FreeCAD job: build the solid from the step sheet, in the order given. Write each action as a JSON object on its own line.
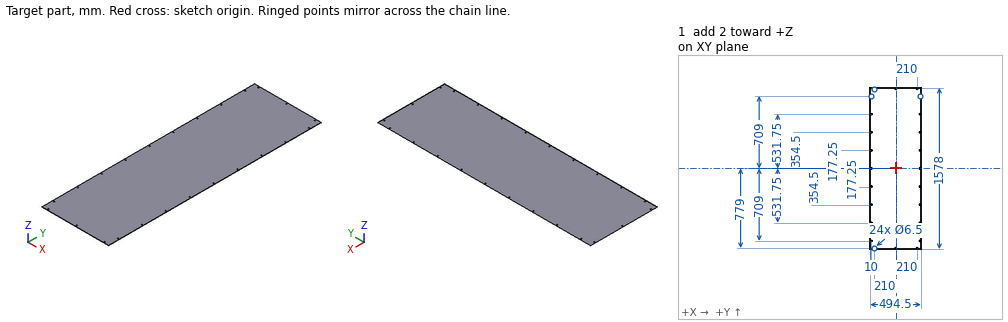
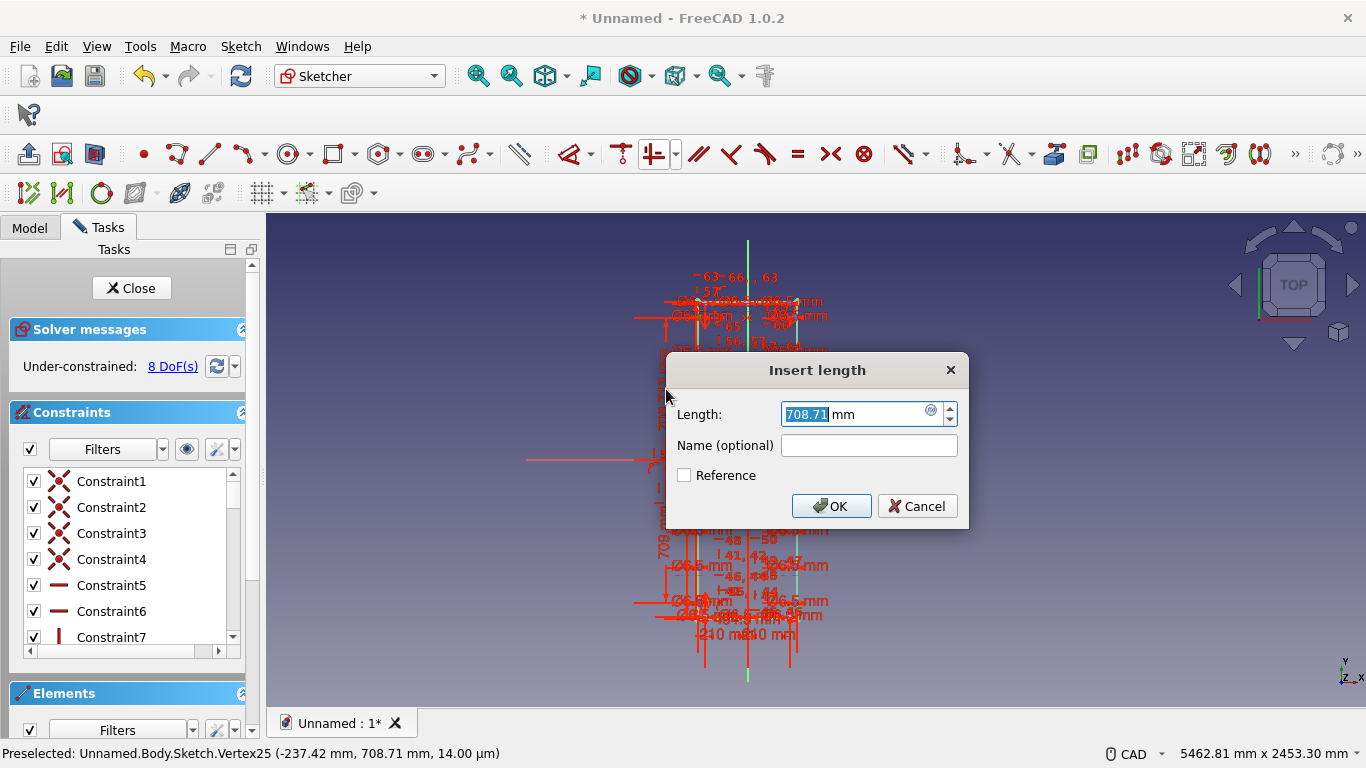
{"action": "type", "text": "709"}
{"action": "key", "text": "Return"}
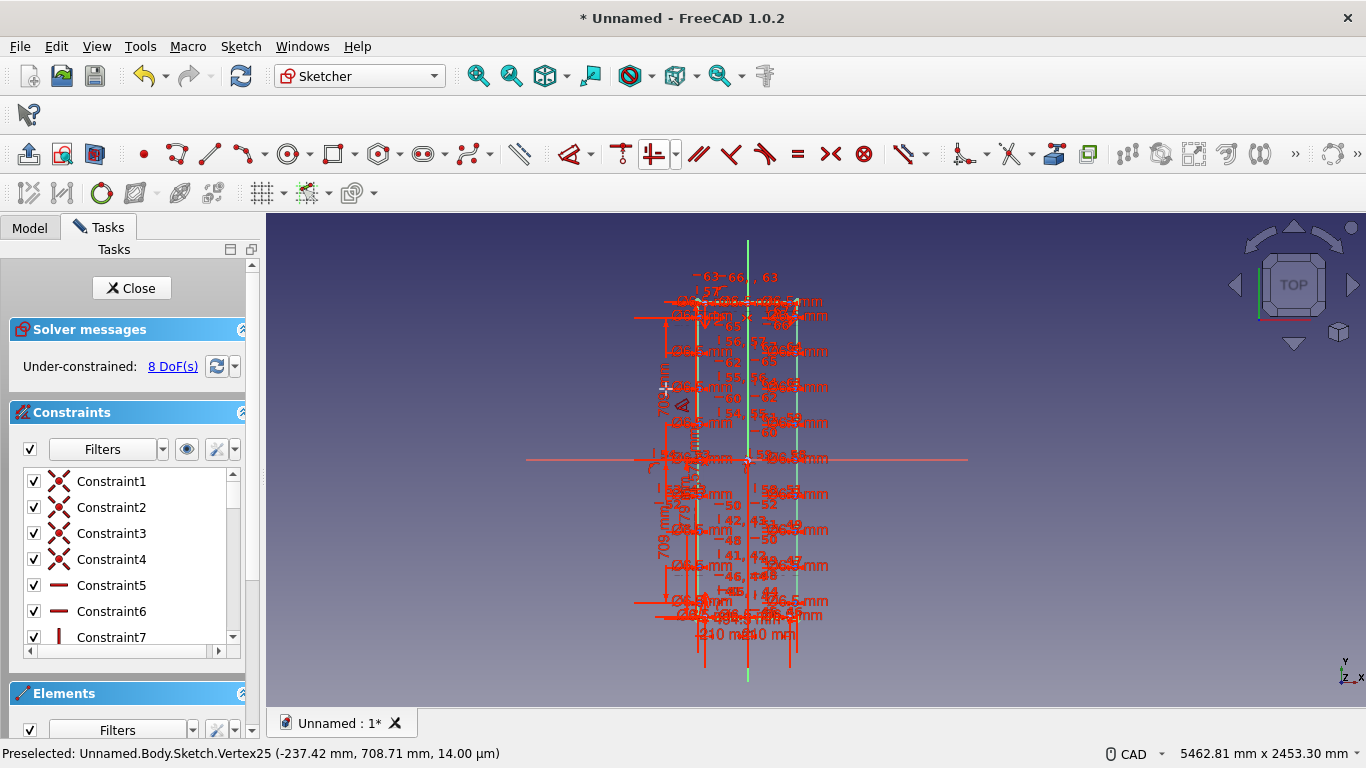
{"action": "scroll", "coordinate": [790, 304], "scroll_direction": "up", "scroll_amount": 3}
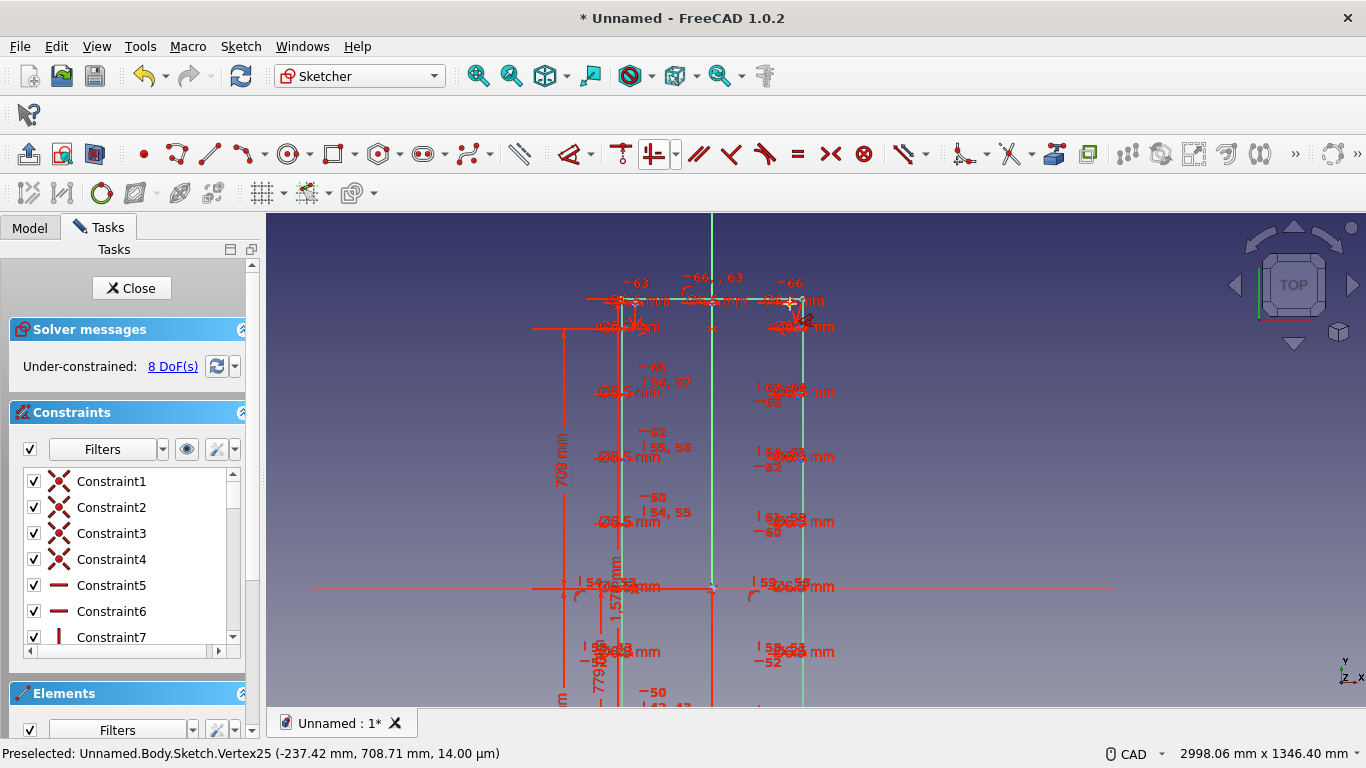
{"action": "left_click", "coordinate": [789, 303]}
{"action": "left_click", "coordinate": [751, 269]}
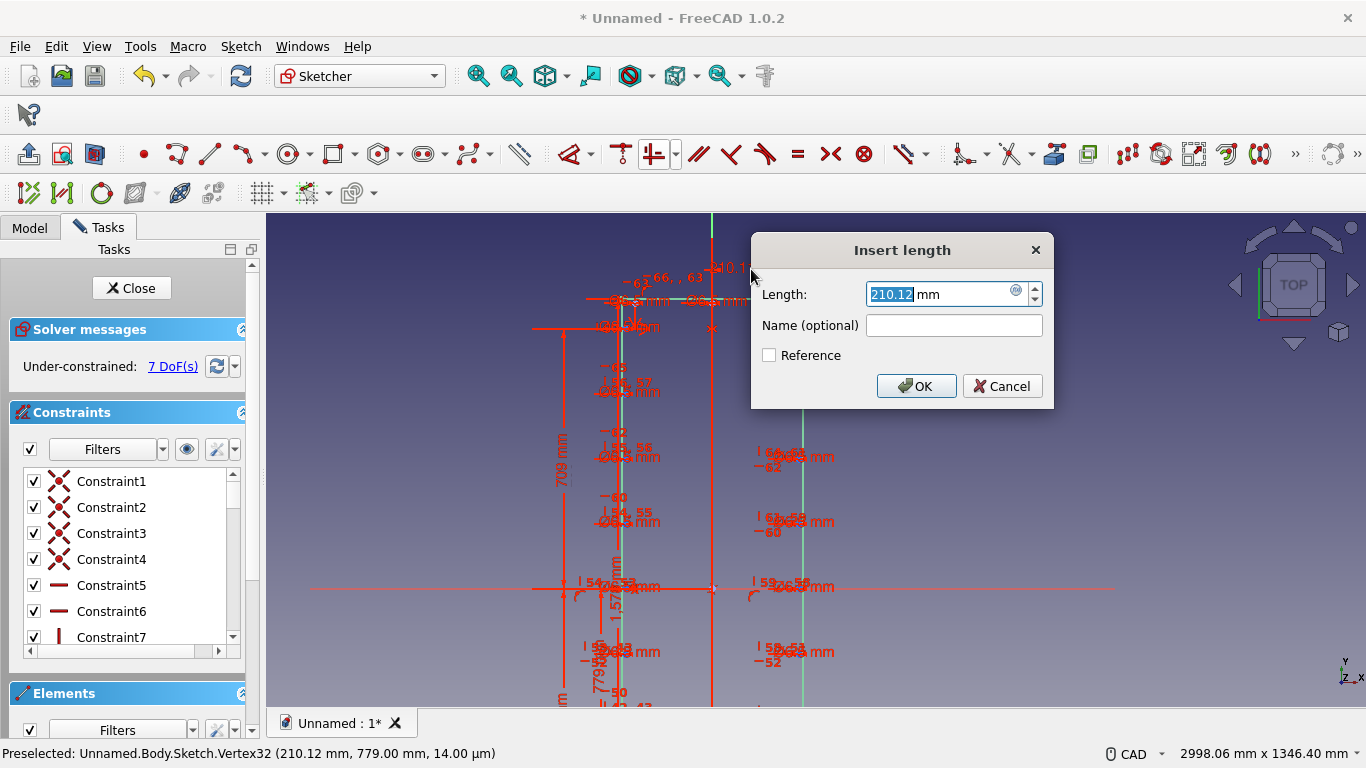
{"action": "type", "text": "210"}
{"action": "key", "text": "Return"}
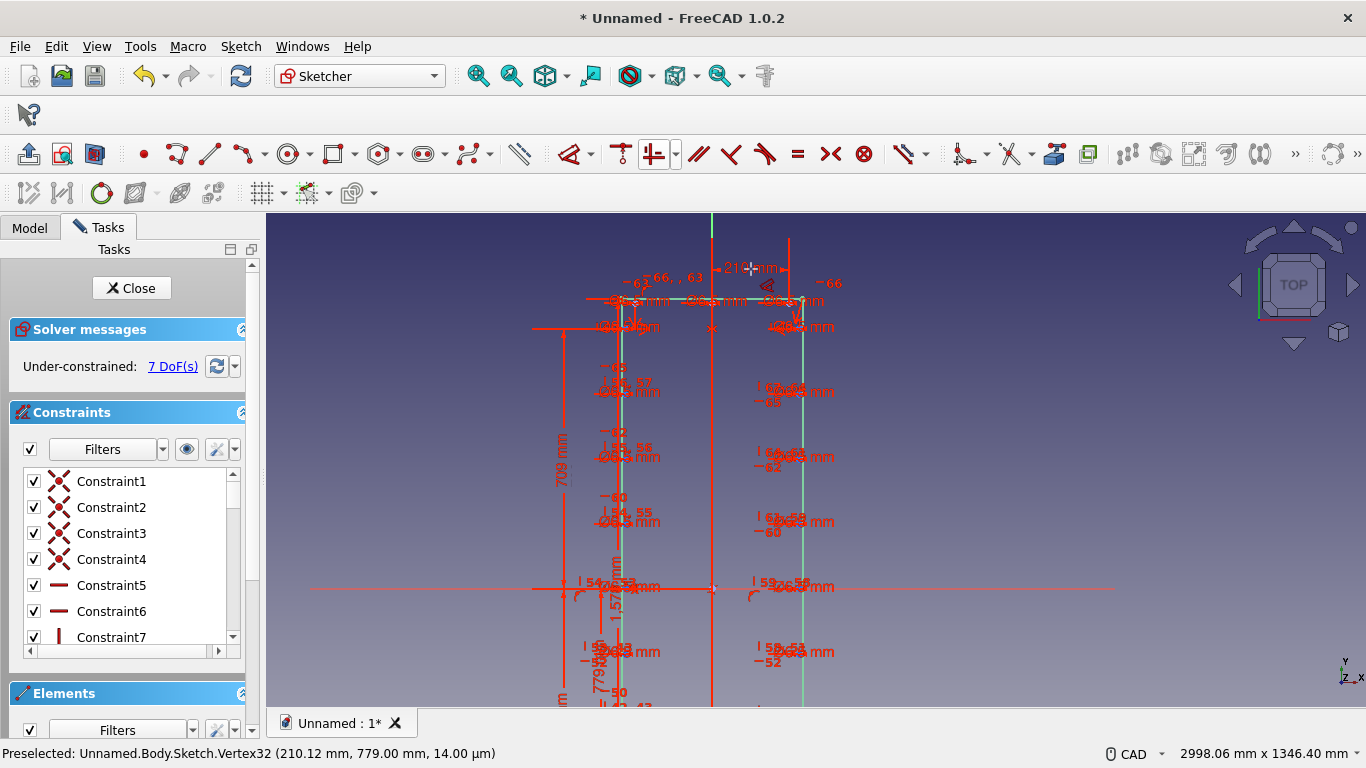
{"action": "scroll", "coordinate": [790, 303], "scroll_direction": "down", "scroll_amount": 3}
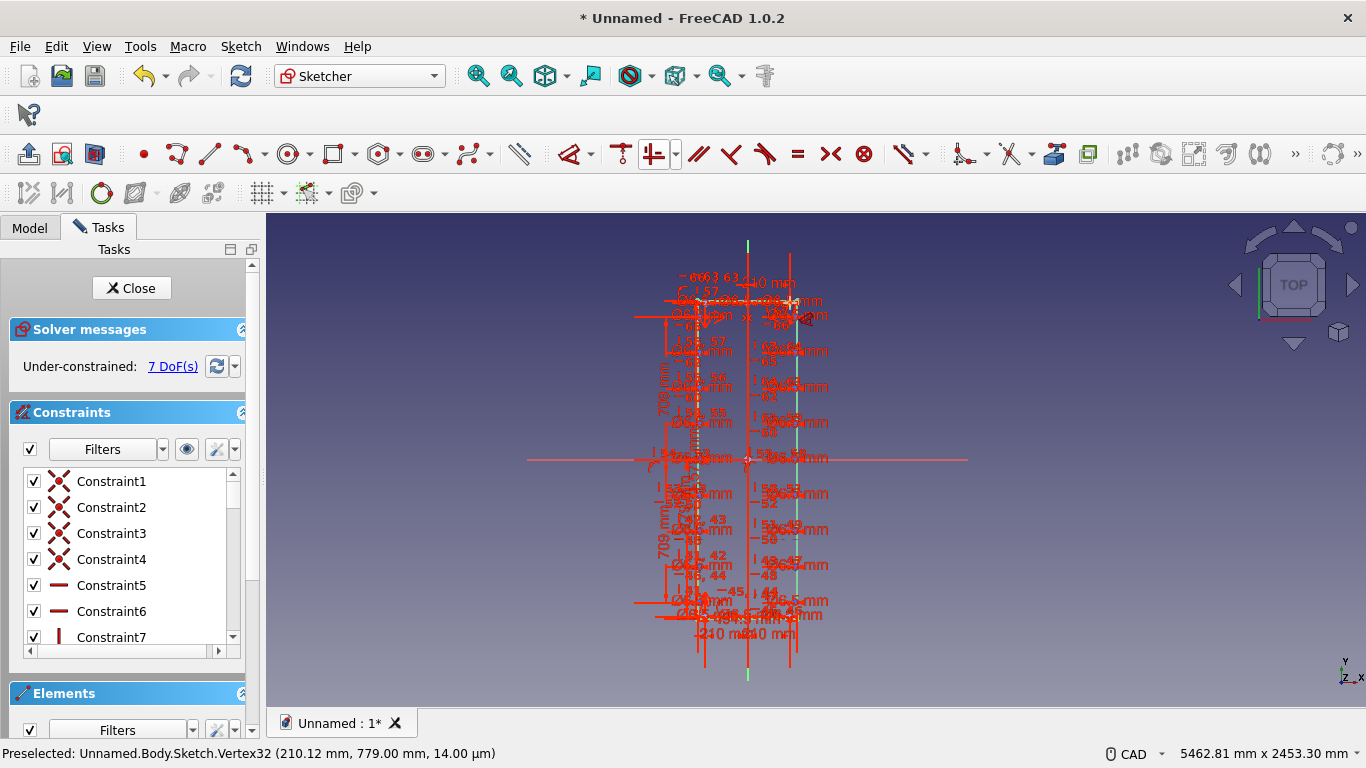
{"action": "scroll", "coordinate": [698, 619], "scroll_direction": "up", "scroll_amount": 15}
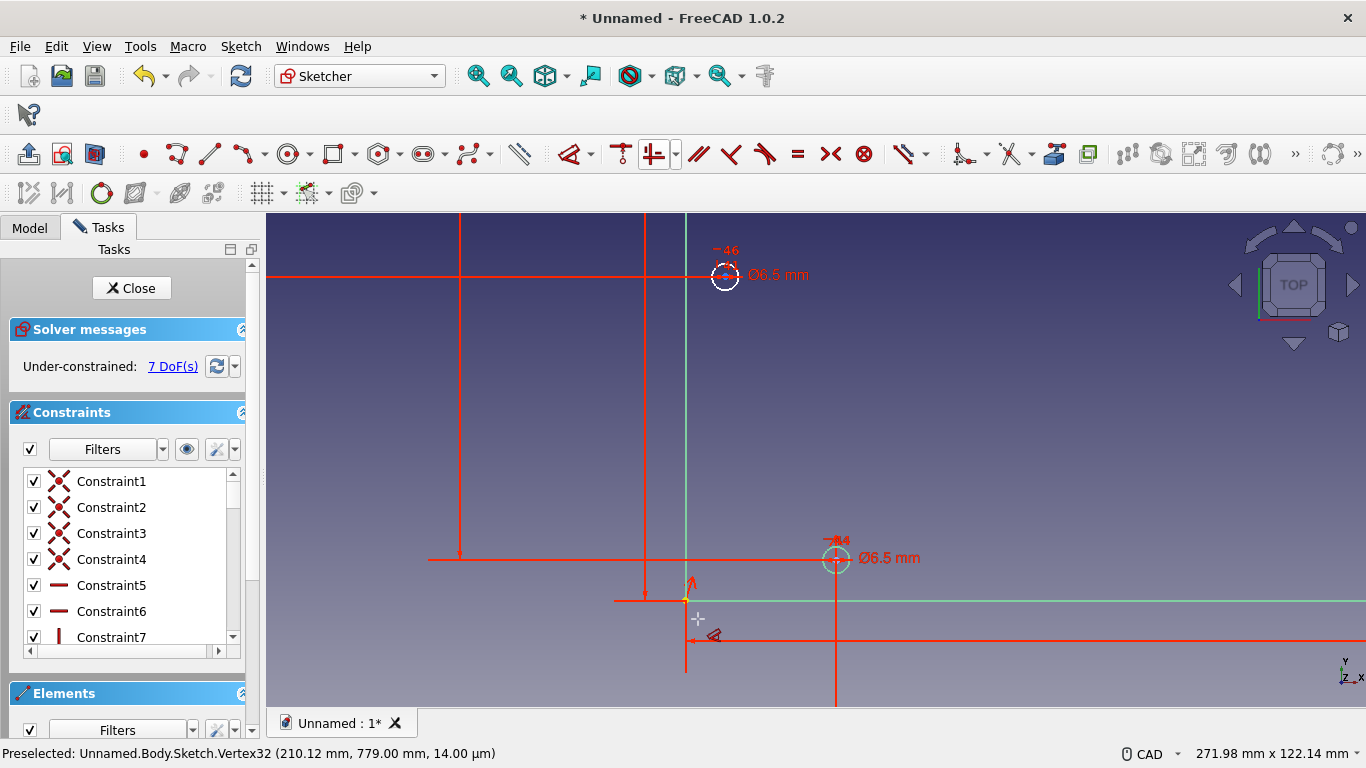
{"action": "left_click", "coordinate": [686, 601]}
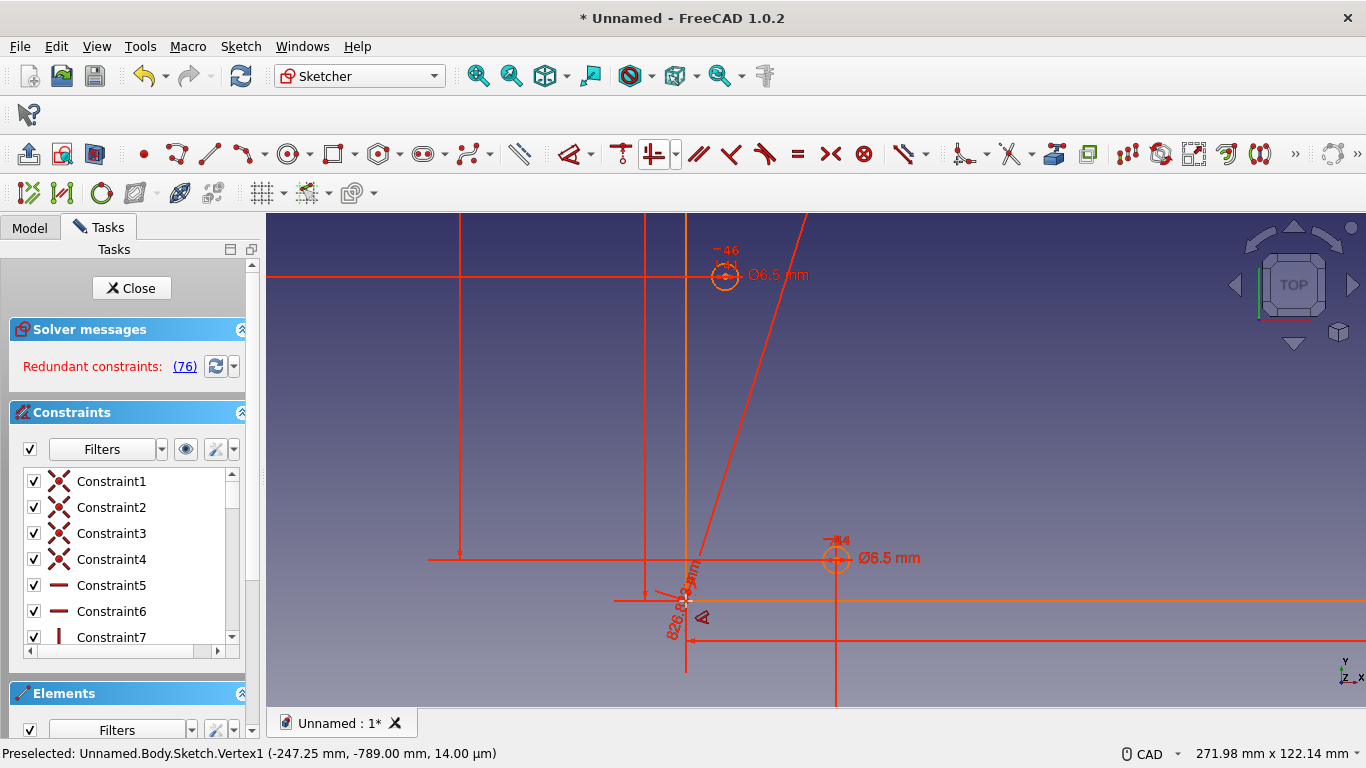
{"action": "left_click", "coordinate": [725, 277]}
{"action": "left_click", "coordinate": [705, 635]}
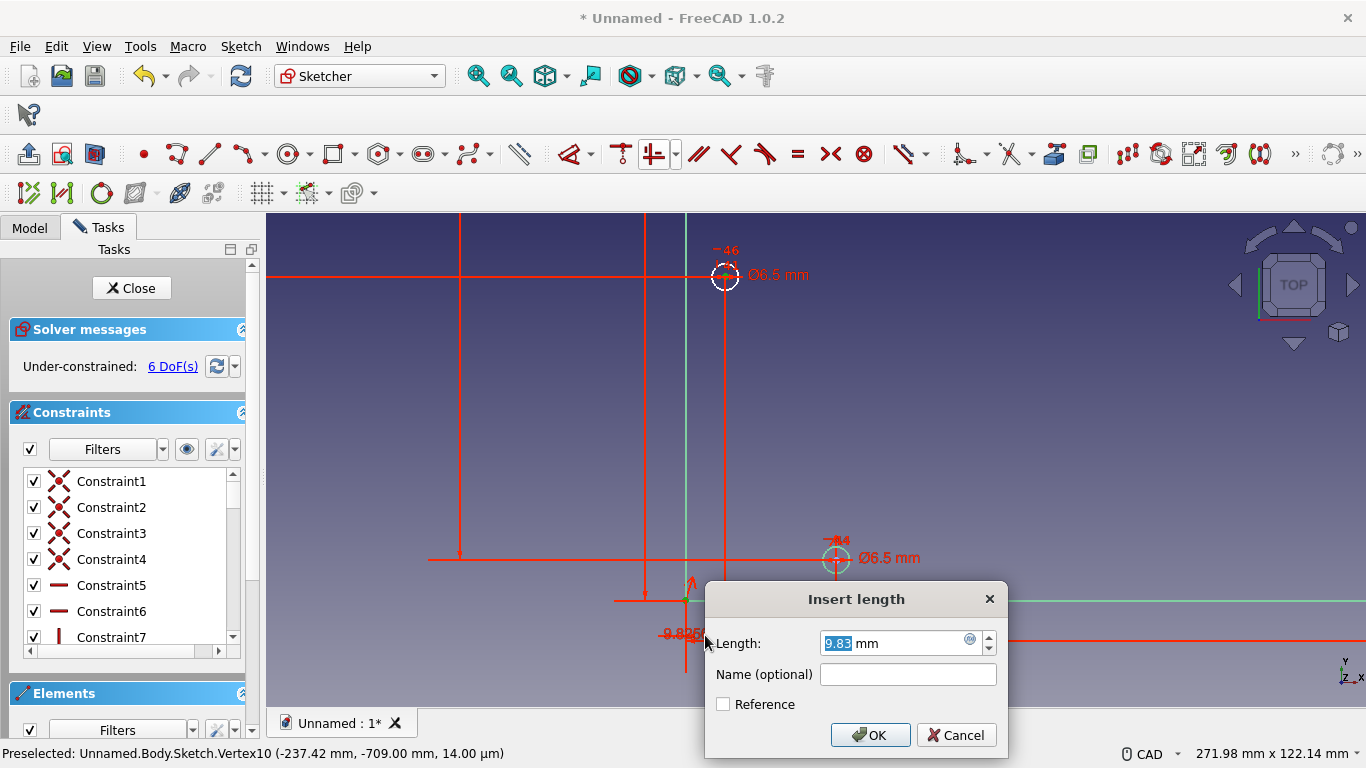
{"action": "type", "text": "10"}
{"action": "key", "text": "Return"}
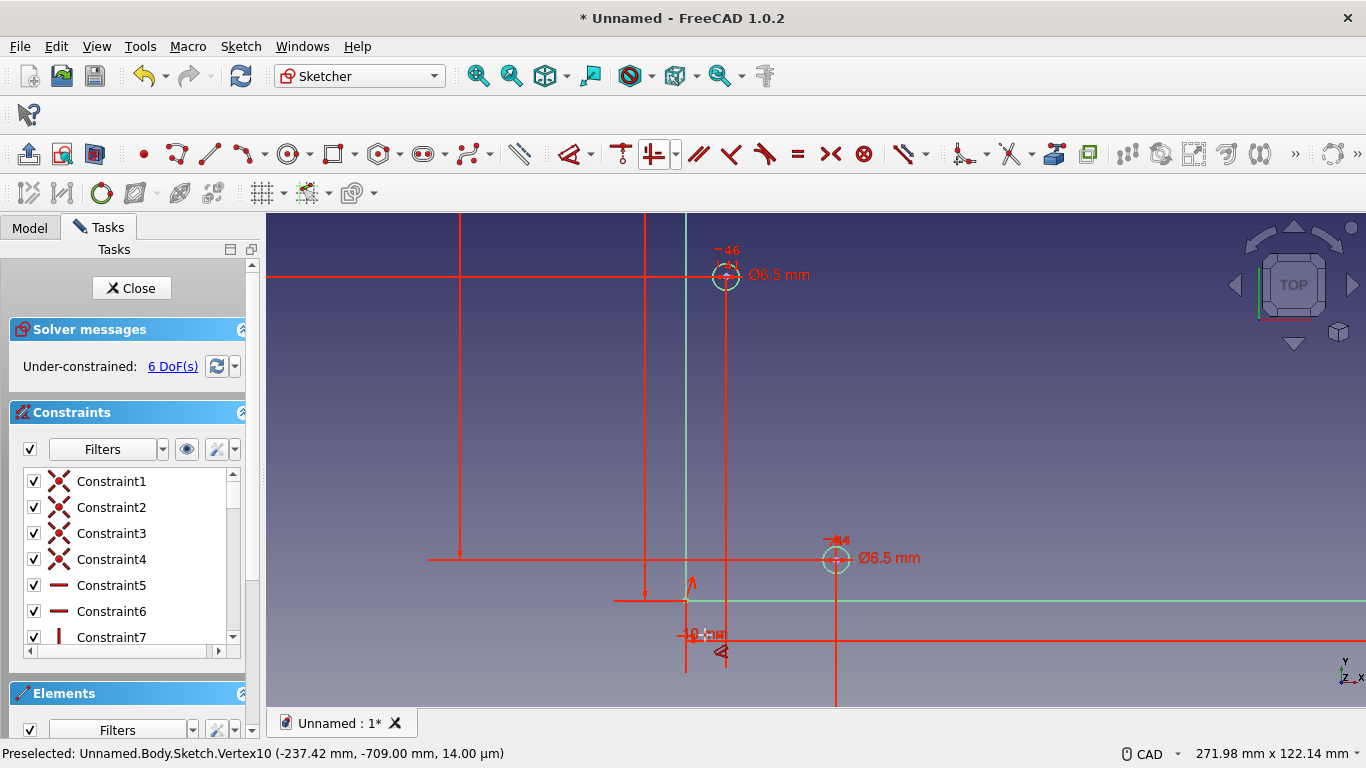
{"action": "scroll", "coordinate": [698, 620], "scroll_direction": "down", "scroll_amount": 15}